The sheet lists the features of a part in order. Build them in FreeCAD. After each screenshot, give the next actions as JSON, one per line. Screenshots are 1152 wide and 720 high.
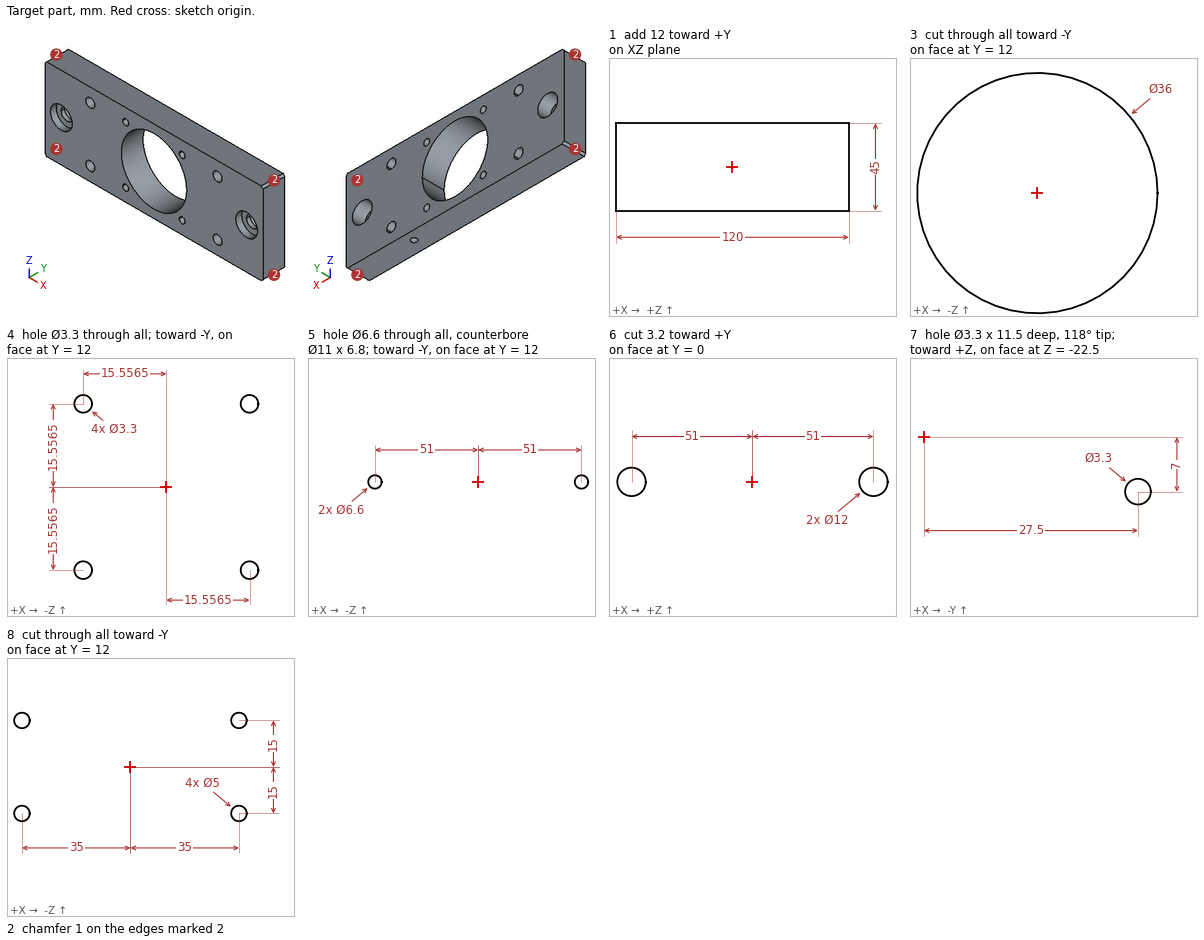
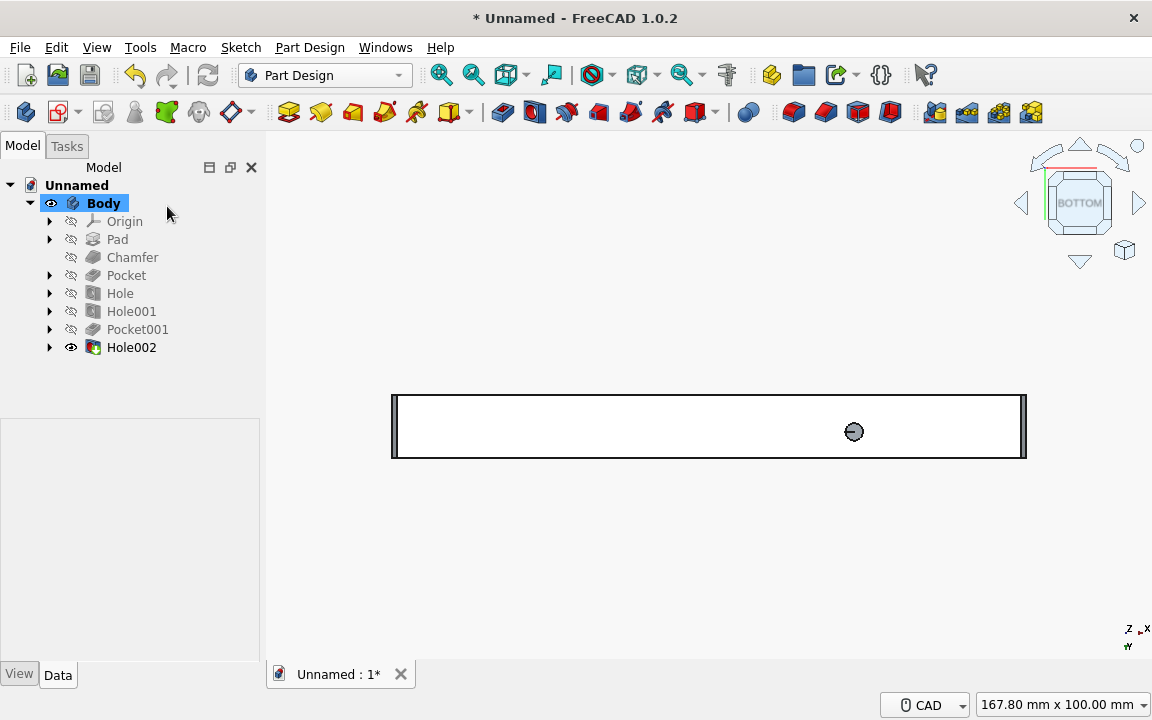
{"action": "key", "text": "4"}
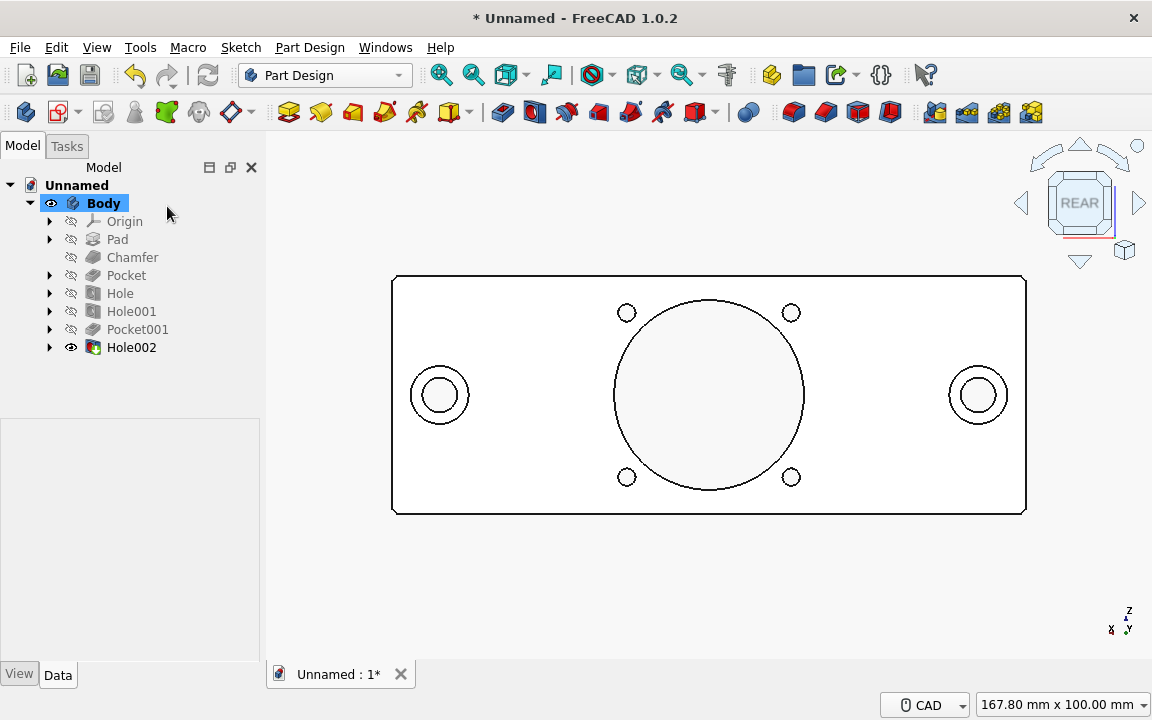
{"action": "left_click", "coordinate": [890, 360]}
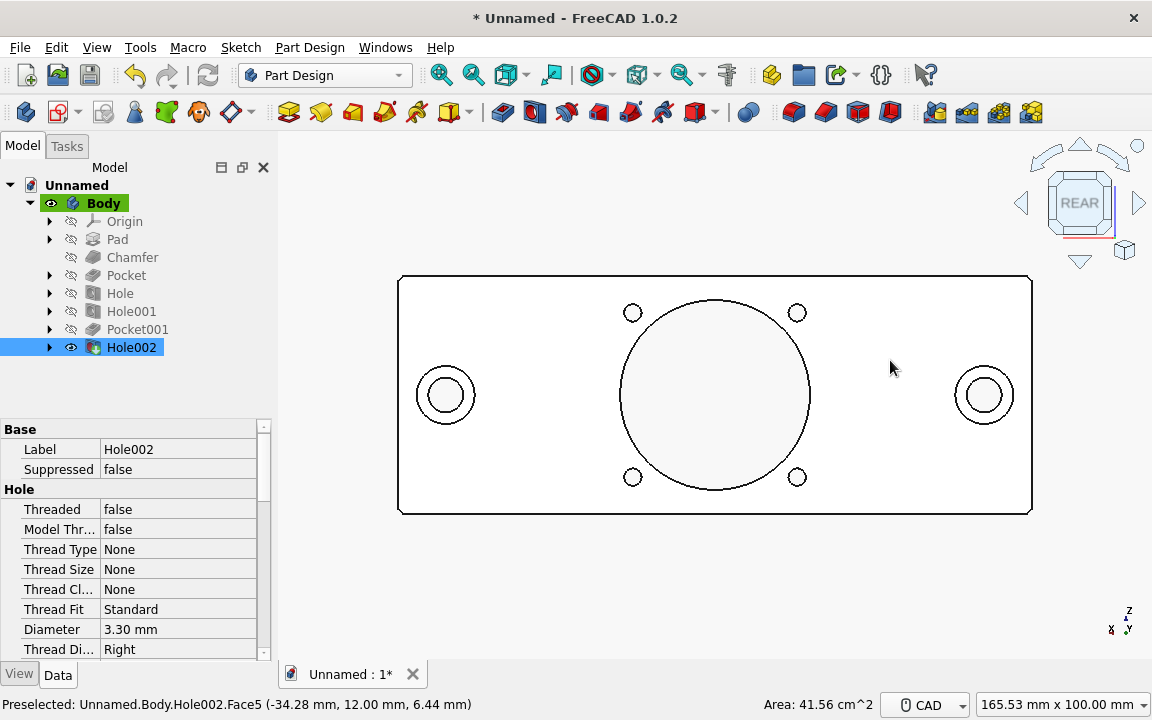
{"action": "left_click", "coordinate": [58, 112]}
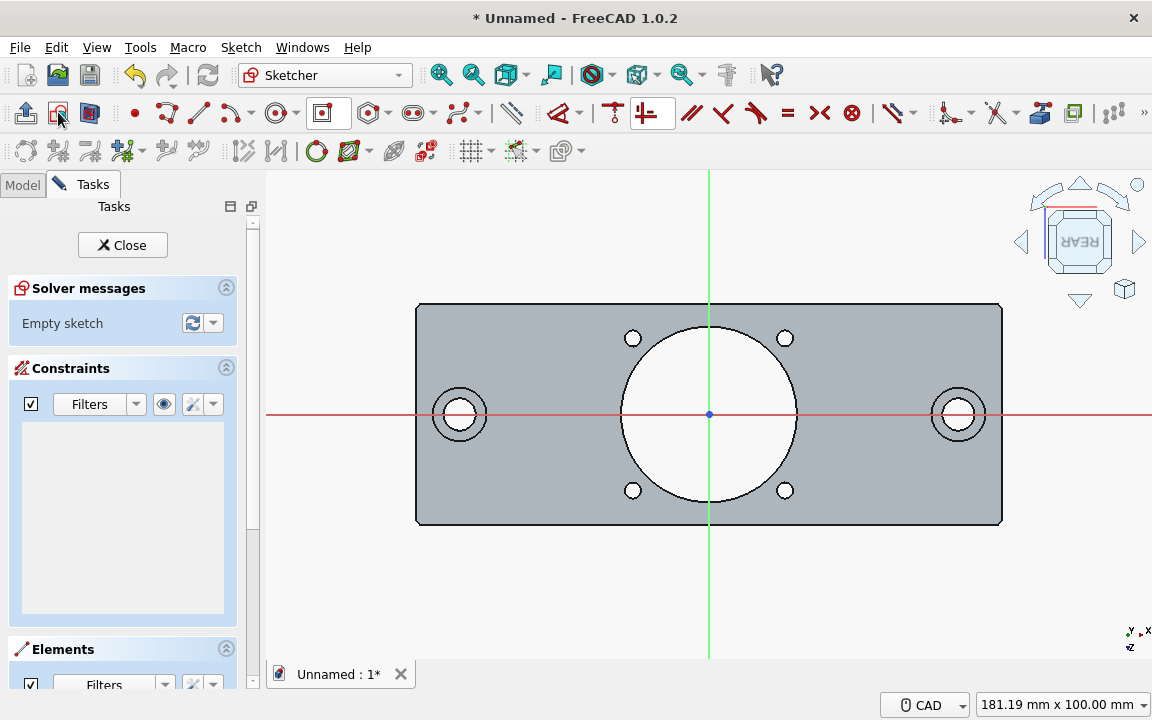
{"action": "left_click", "coordinate": [276, 114]}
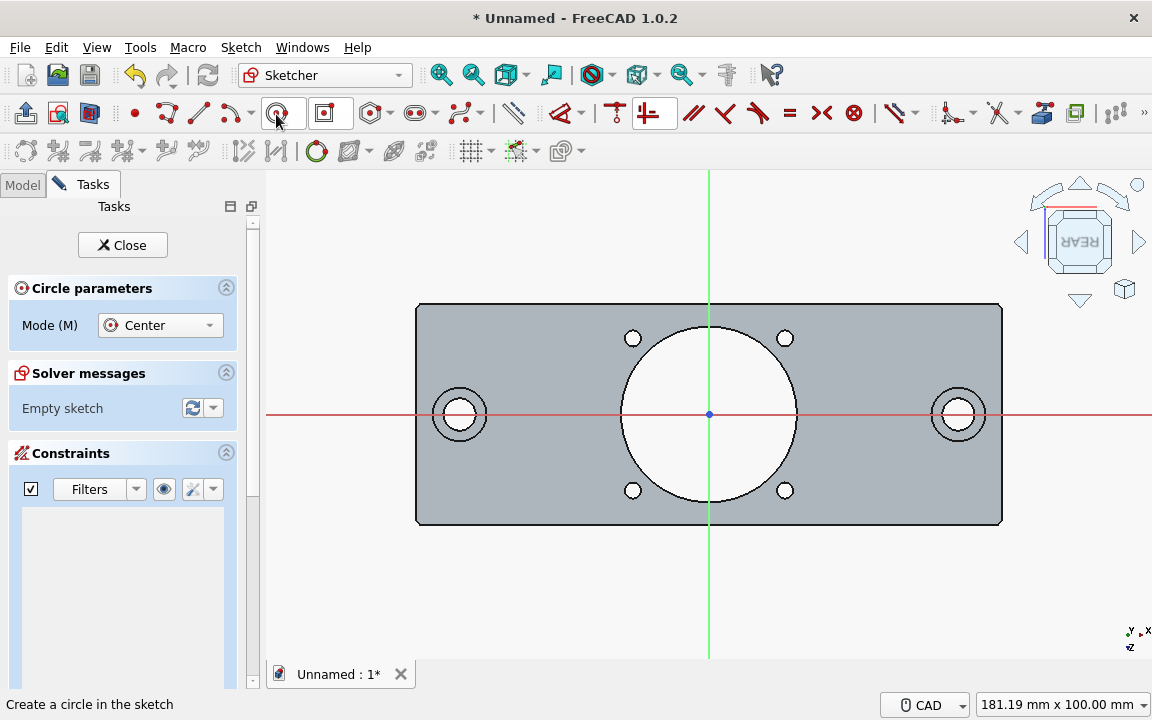
{"action": "scroll", "coordinate": [880, 488], "scroll_direction": "up", "scroll_amount": 4}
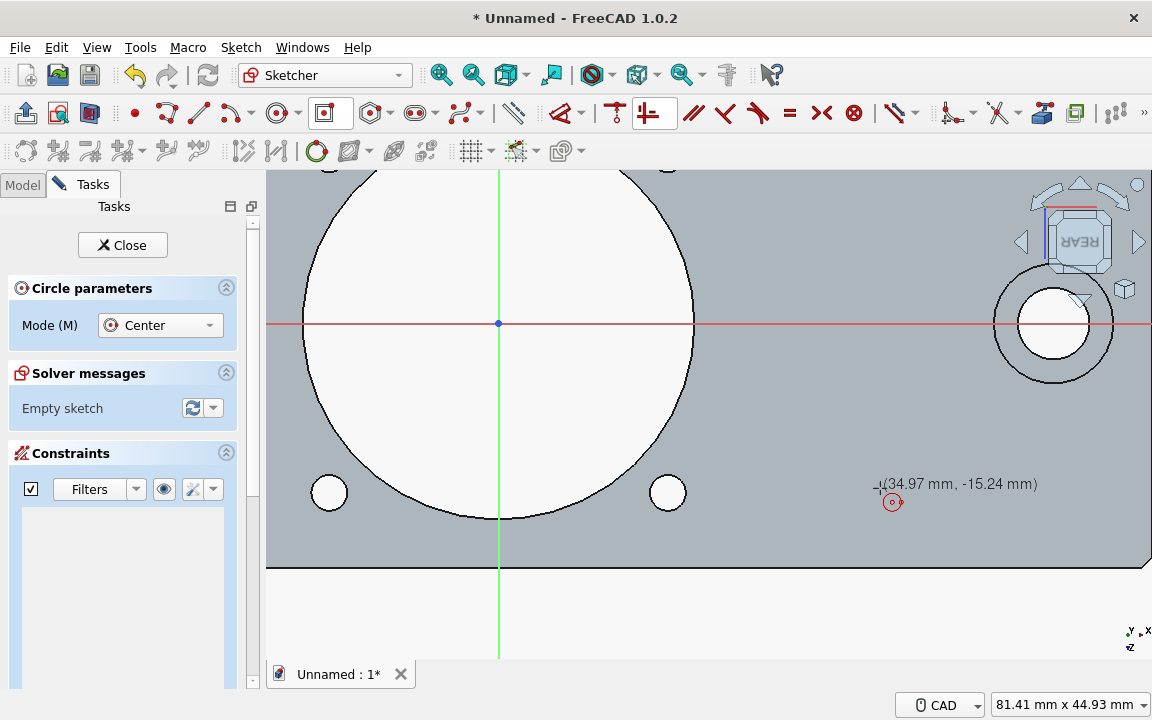
{"action": "left_click", "coordinate": [879, 487]}
{"action": "mouse_move", "coordinate": [899, 468]}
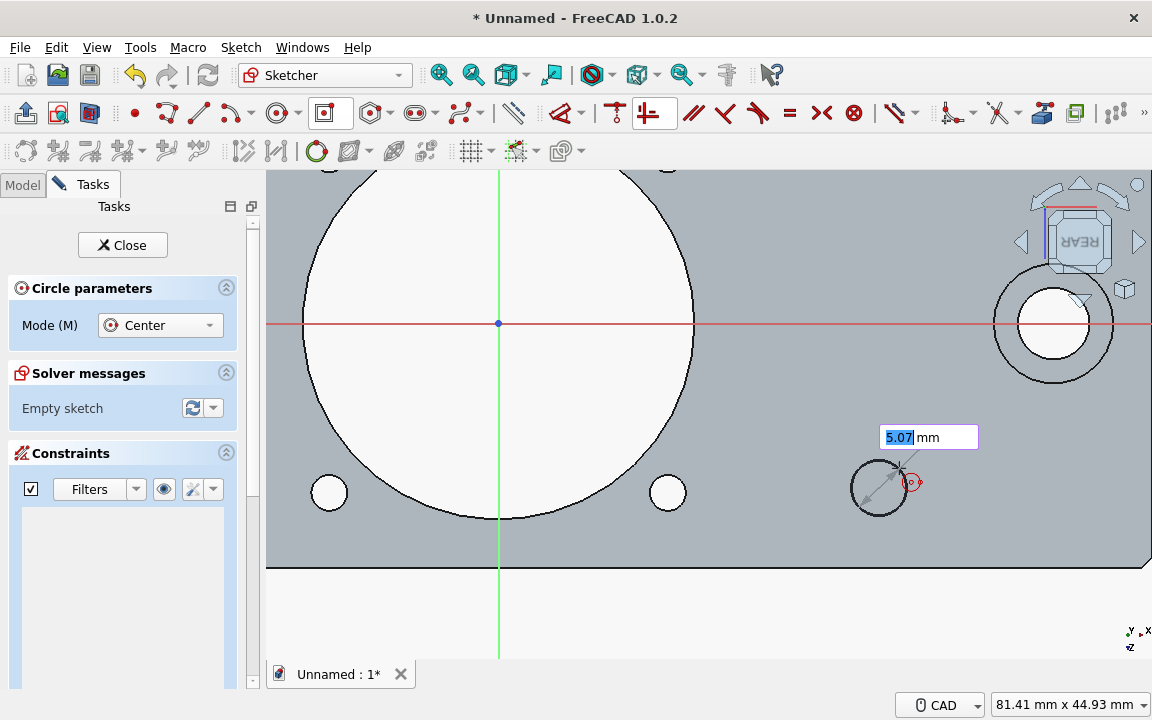
{"action": "type", "text": "5"}
{"action": "key", "text": "Return"}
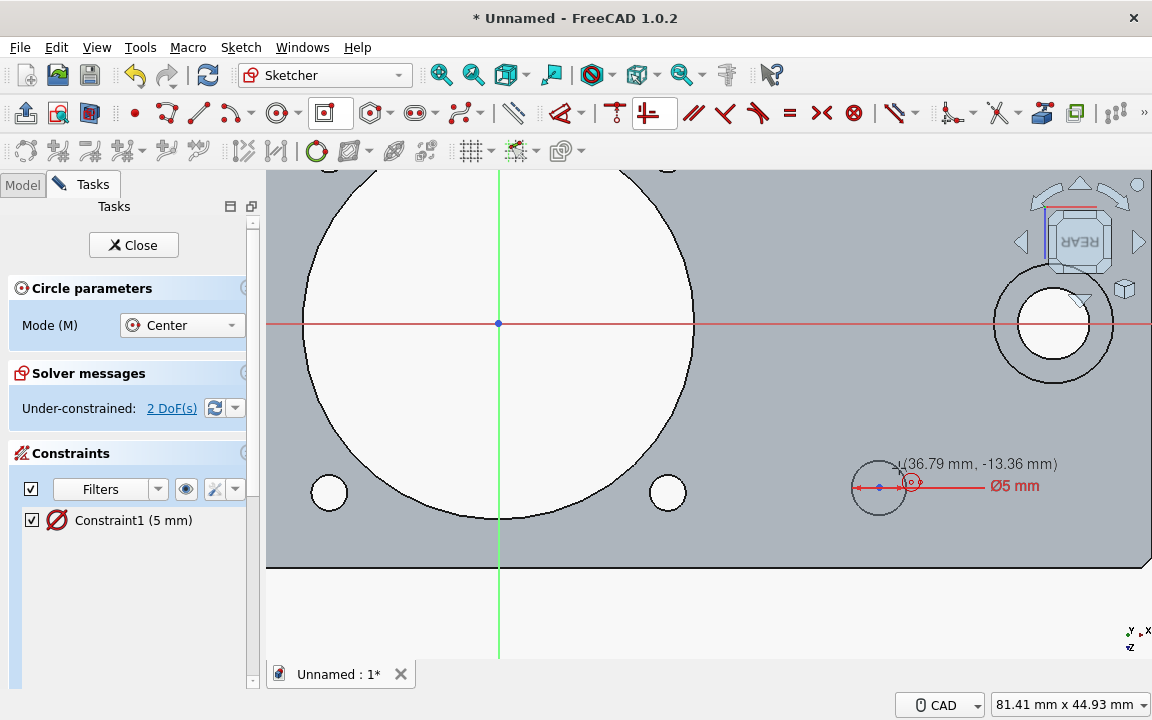
{"action": "scroll", "coordinate": [813, 525], "scroll_direction": "down", "scroll_amount": 3}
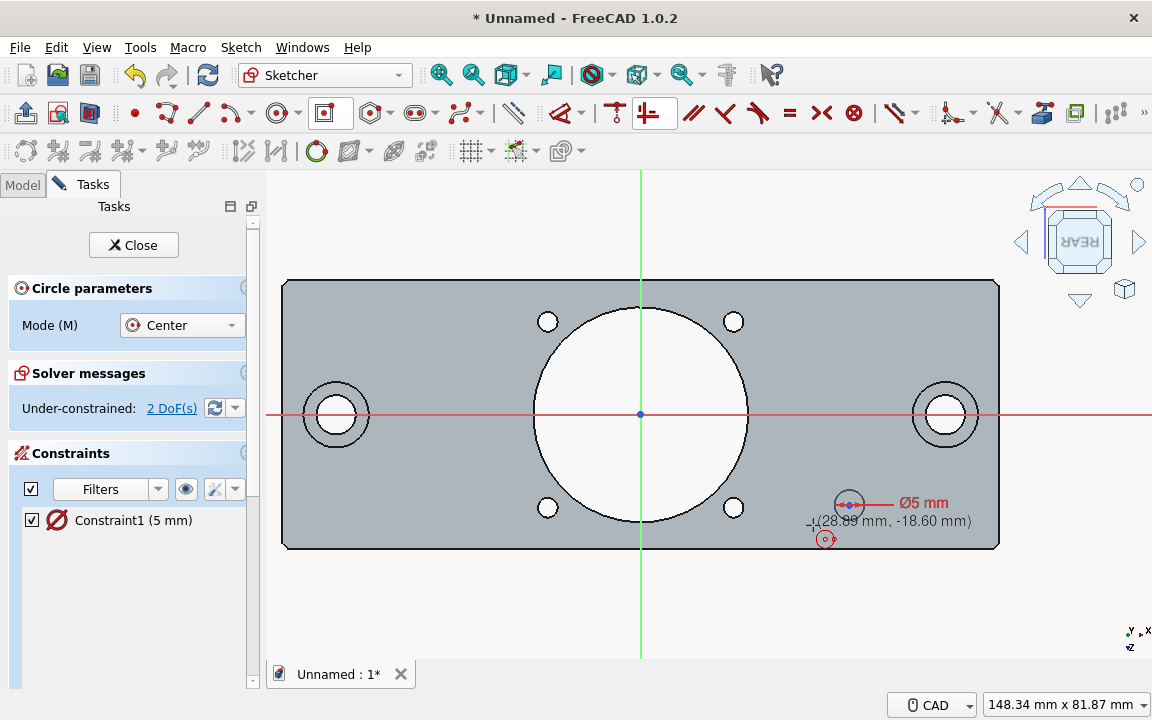
{"action": "scroll", "coordinate": [850, 325], "scroll_direction": "up", "scroll_amount": 3}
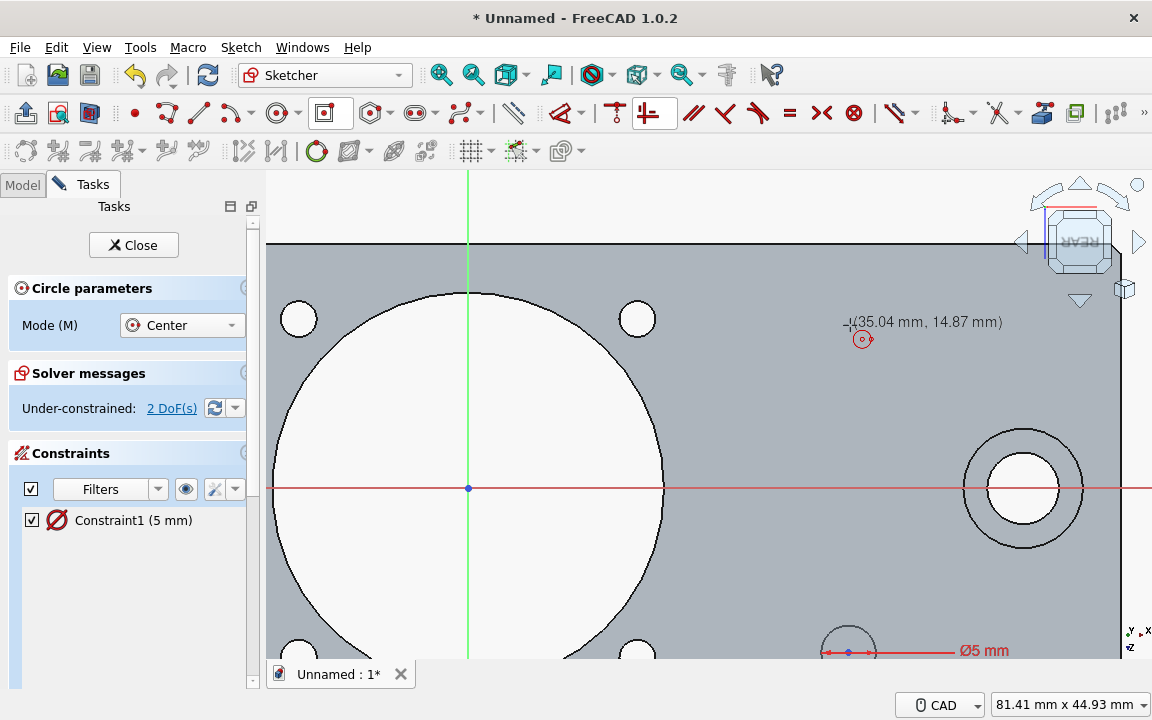
{"action": "left_click", "coordinate": [849, 325]}
{"action": "mouse_move", "coordinate": [868, 306]}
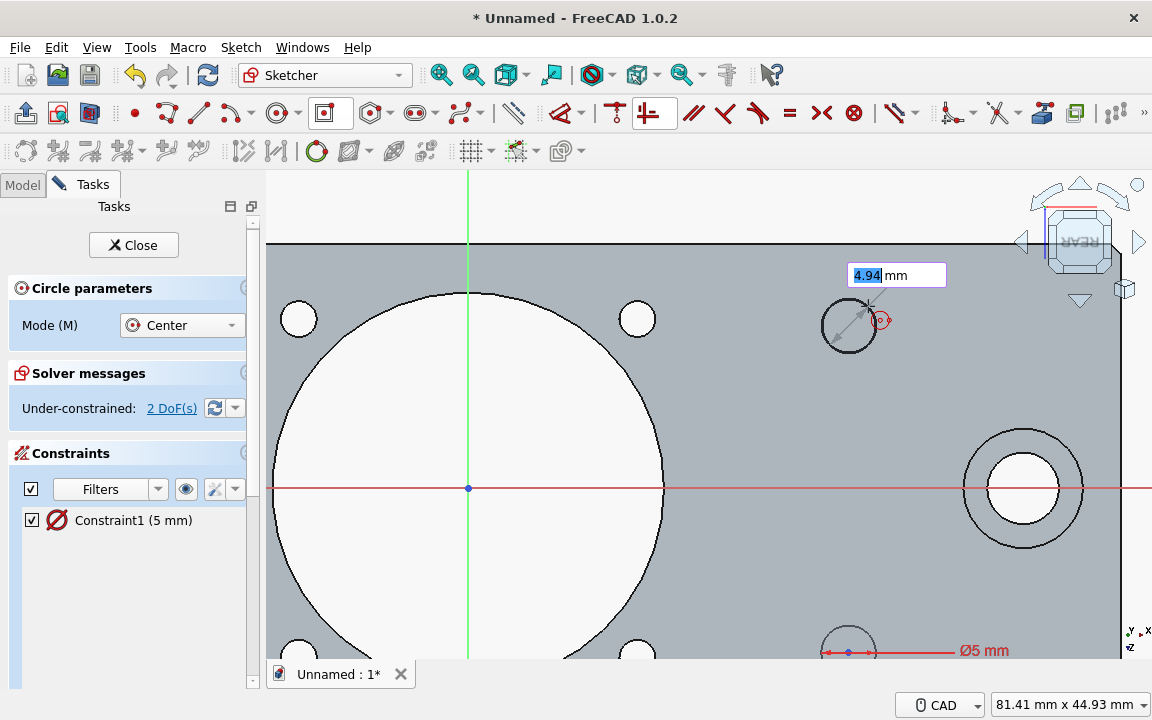
{"action": "type", "text": "5"}
{"action": "key", "text": "Return"}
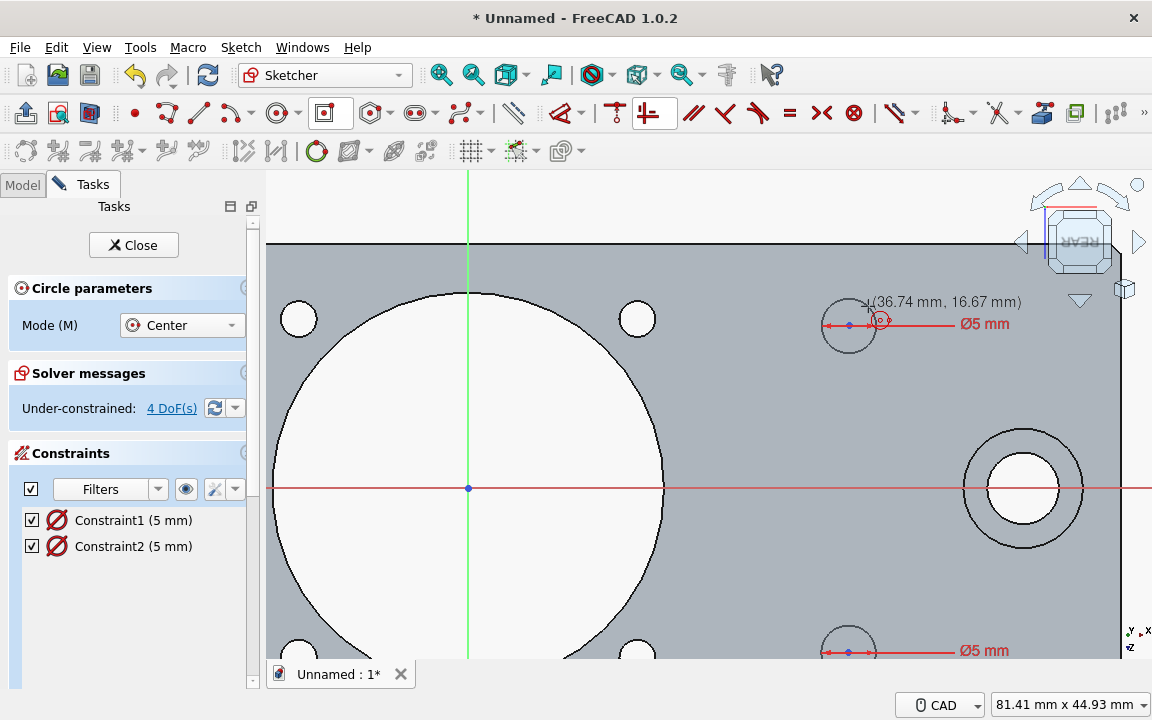
{"action": "scroll", "coordinate": [850, 325], "scroll_direction": "down", "scroll_amount": 3}